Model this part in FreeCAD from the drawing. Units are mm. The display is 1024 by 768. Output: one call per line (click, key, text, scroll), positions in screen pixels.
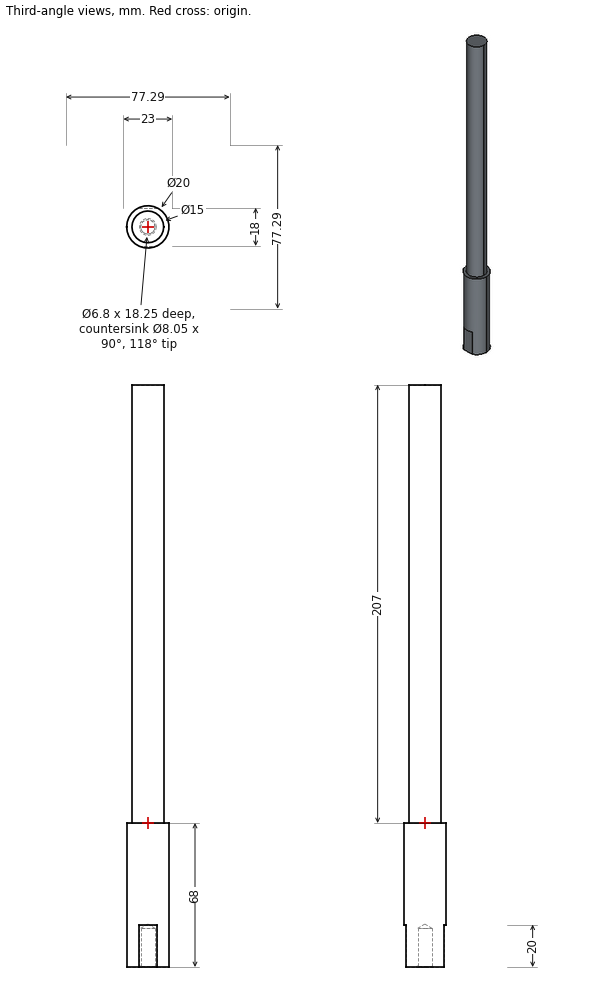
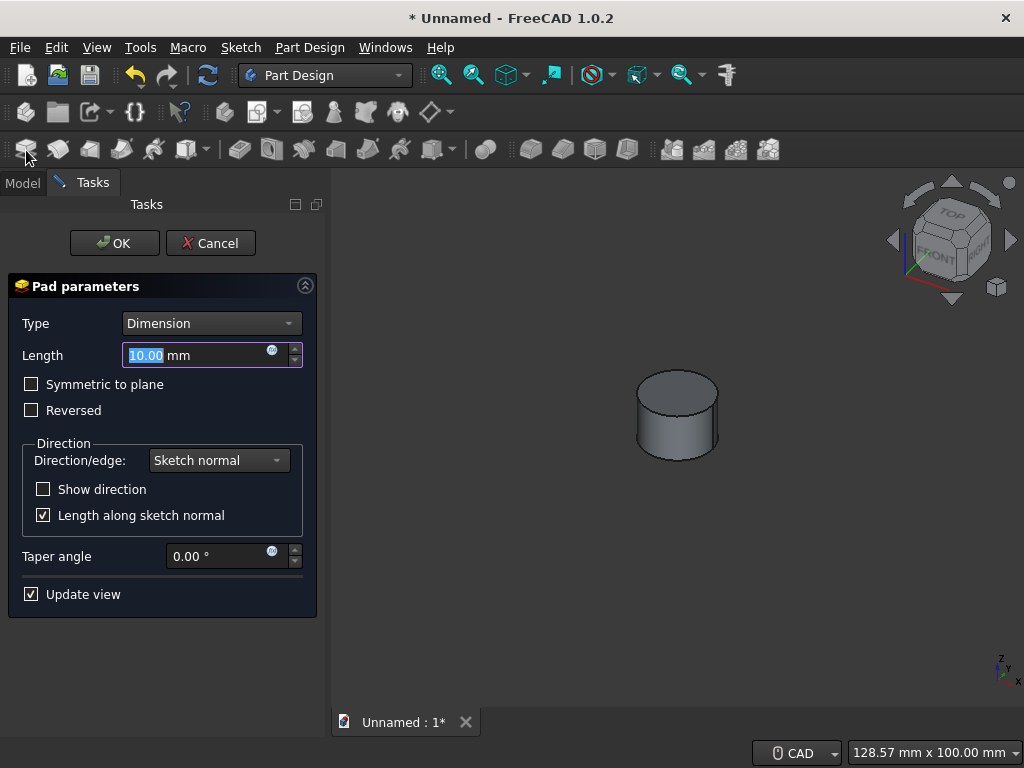
text(207)
key(Tab)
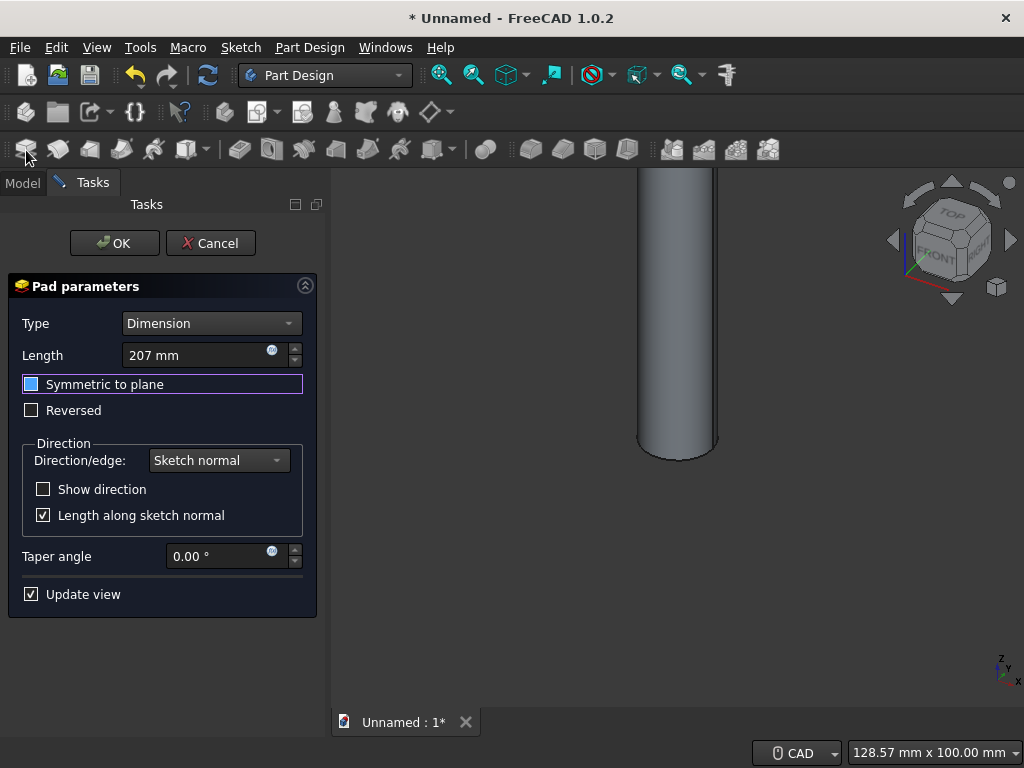
click(115, 243)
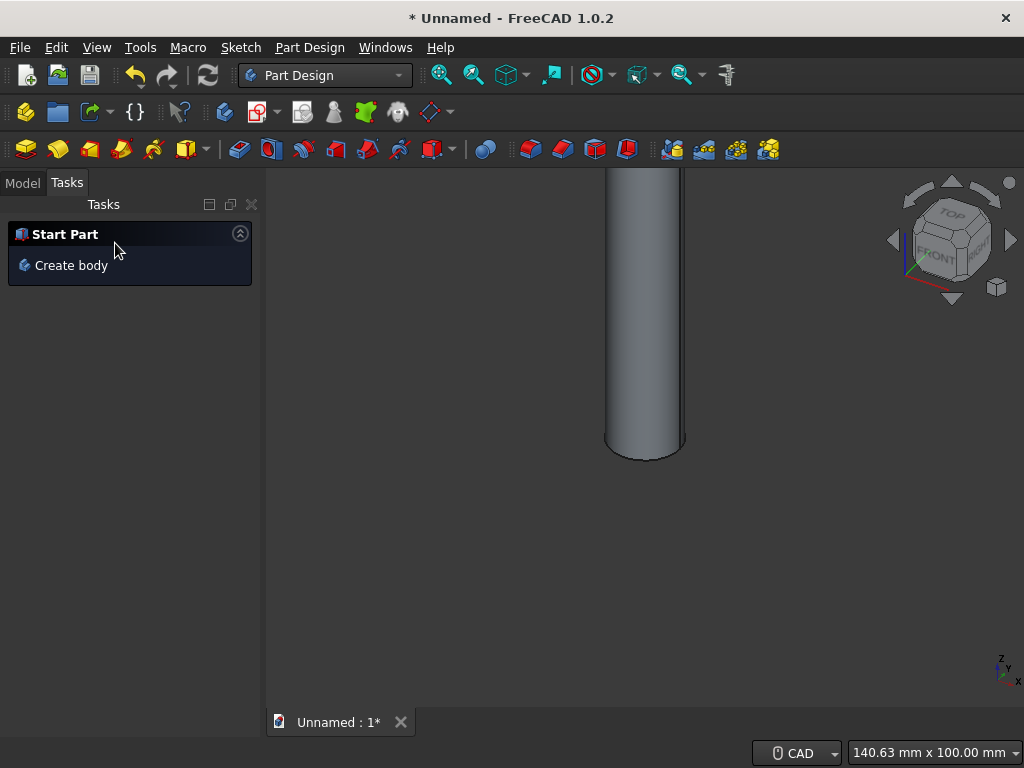
click(442, 76)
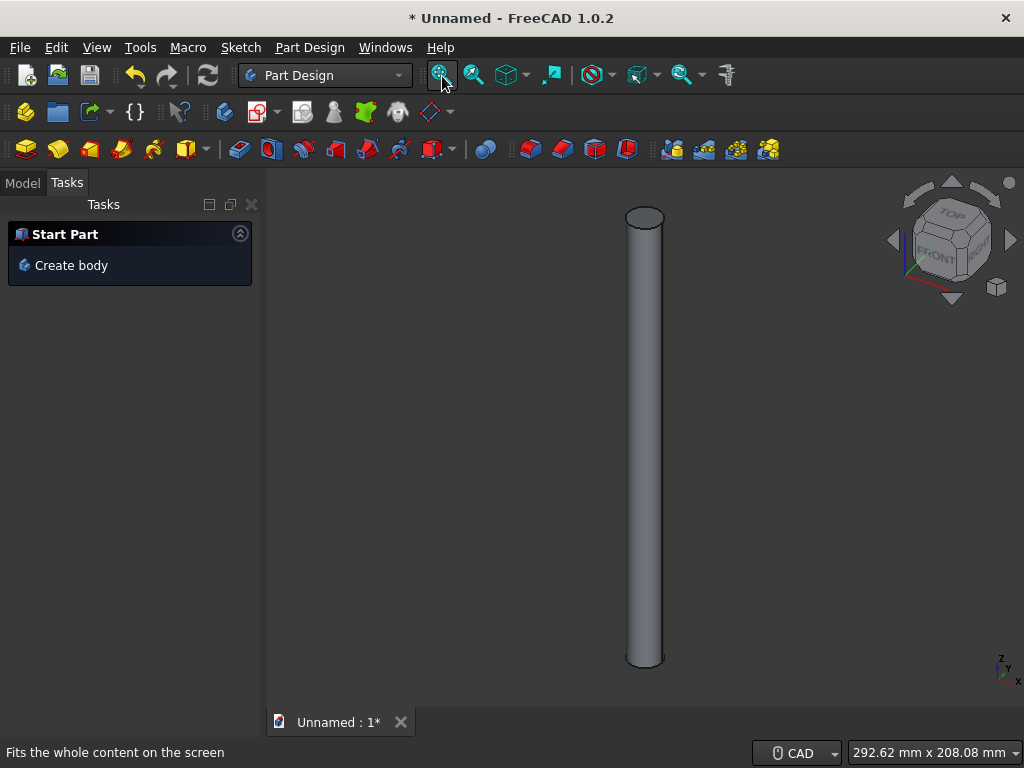
click(258, 112)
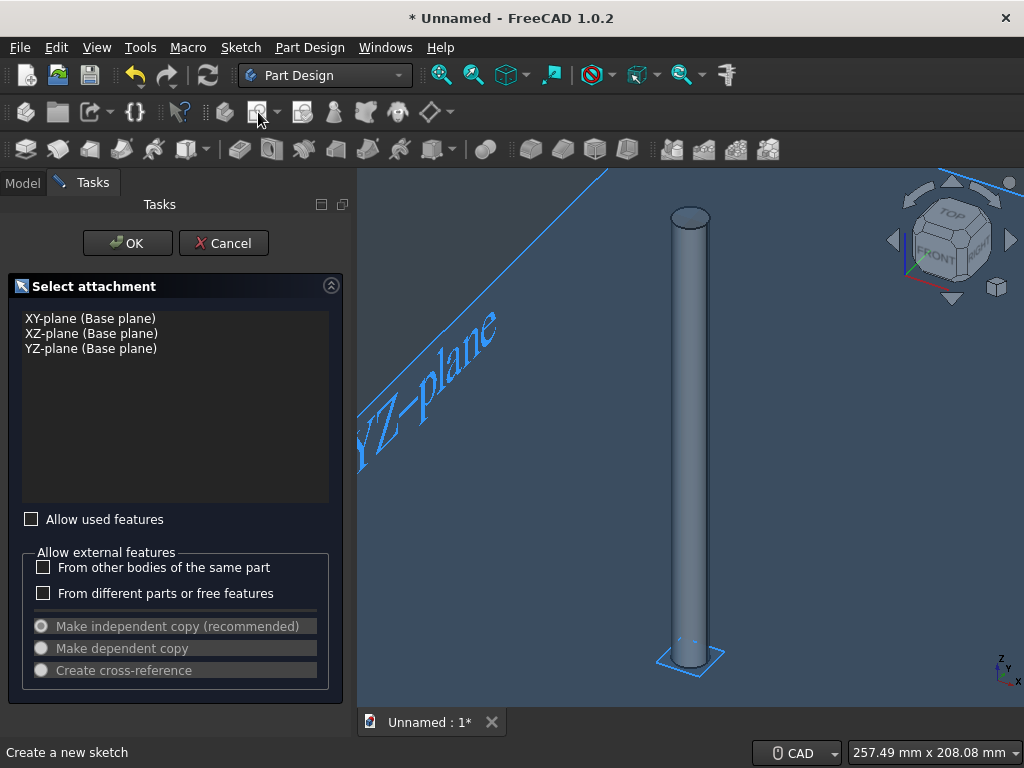
click(82, 318)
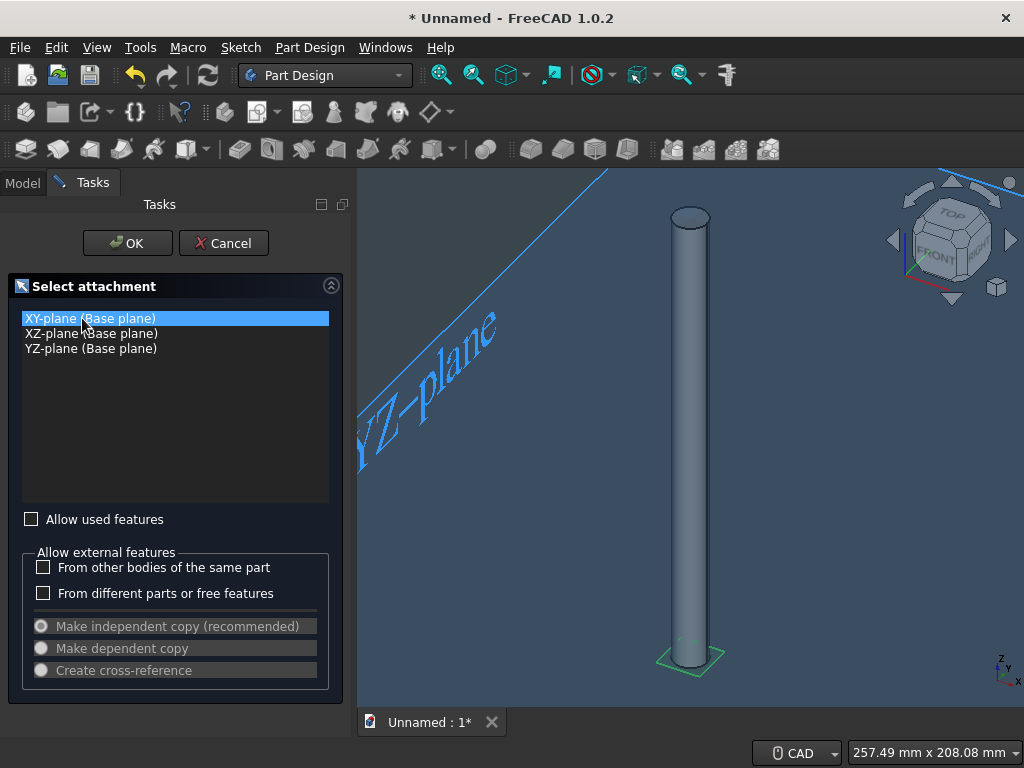
click(128, 243)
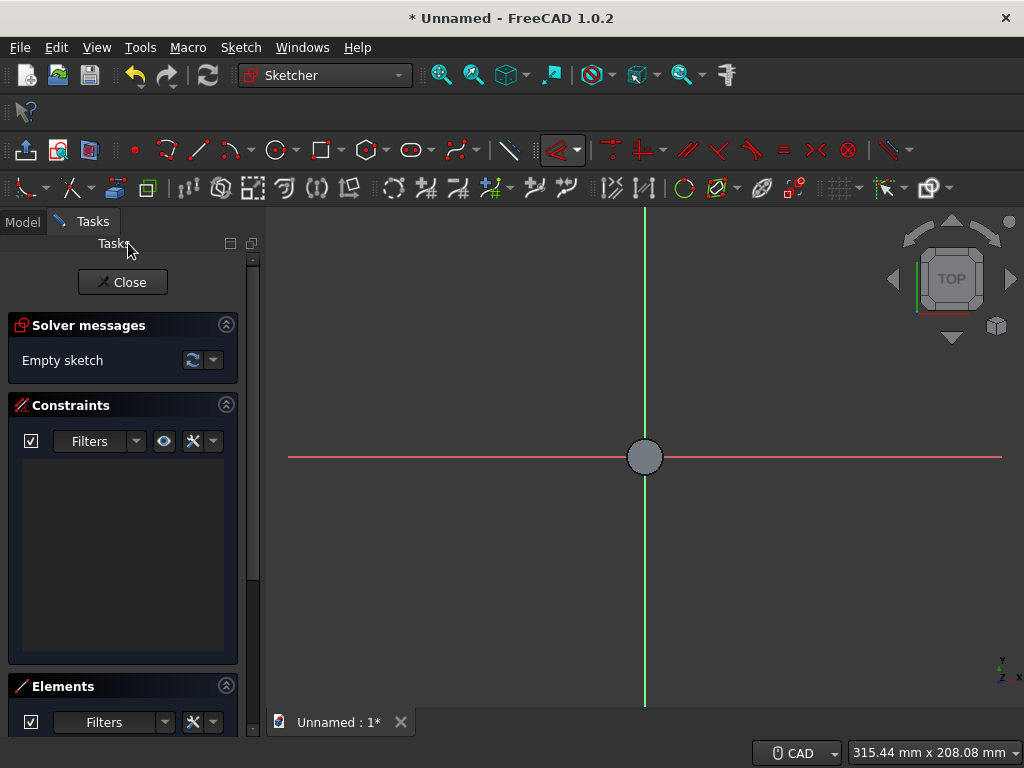
click(90, 150)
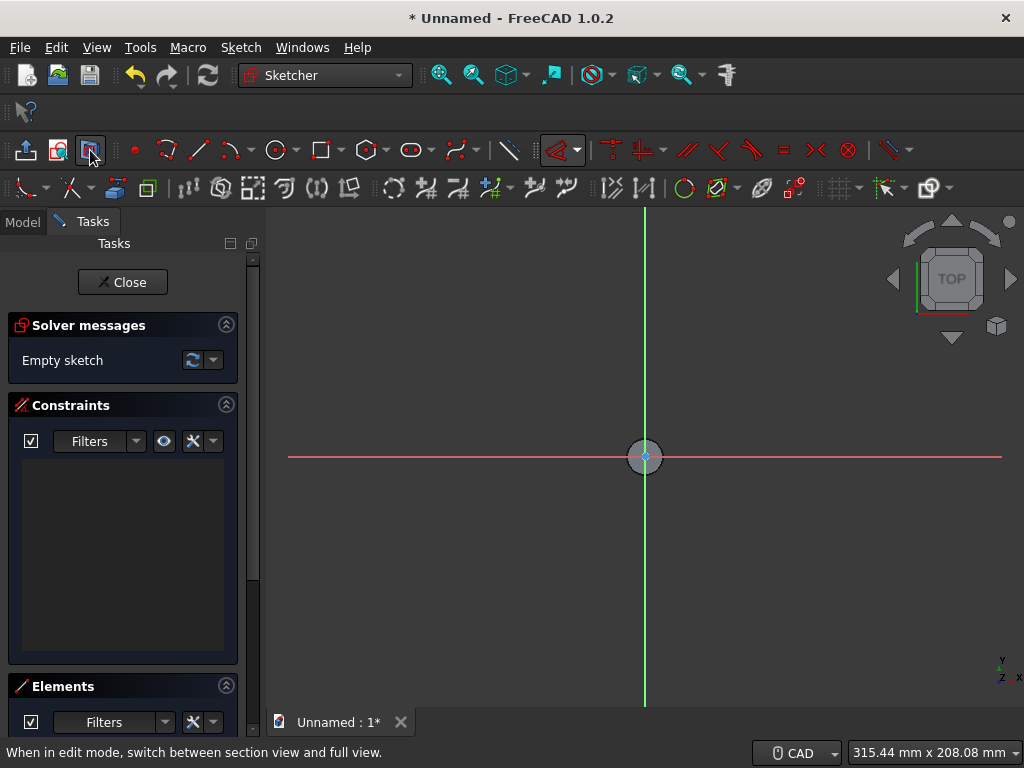
scroll(659, 457, up, 9)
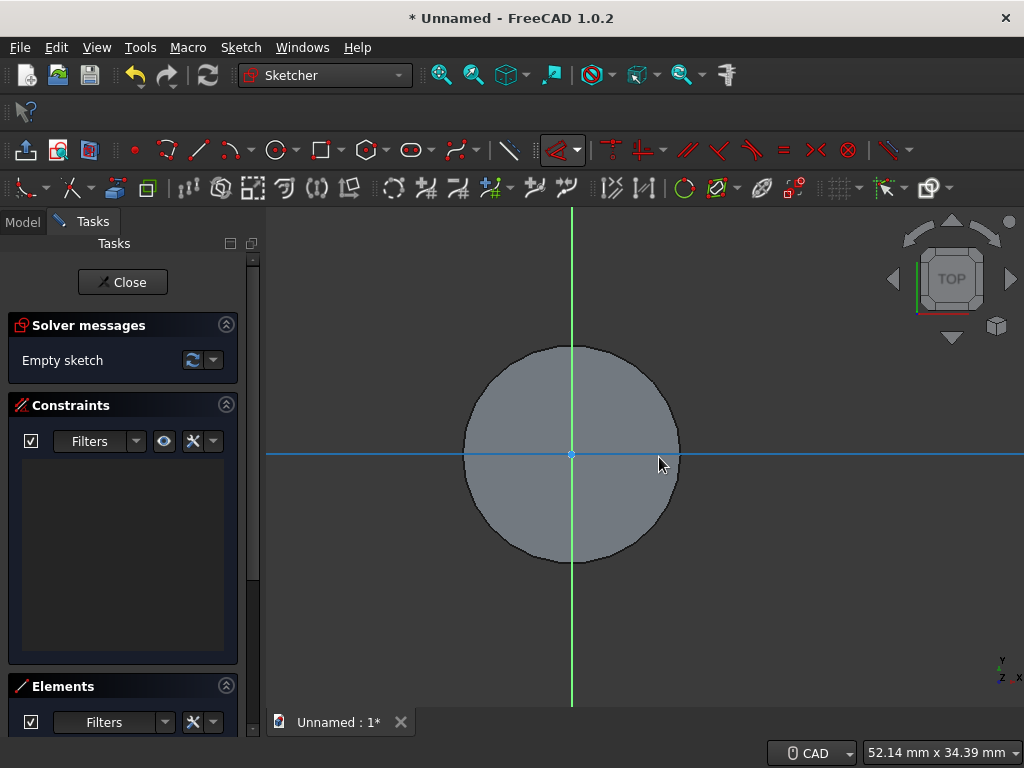
click(276, 150)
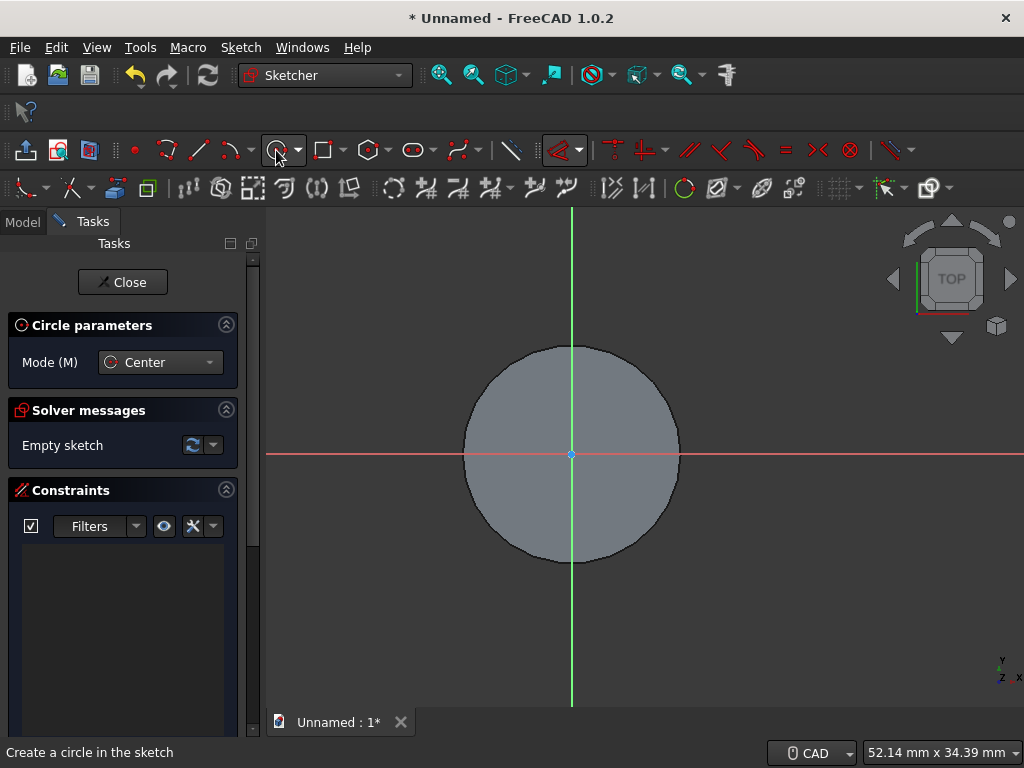
click(572, 454)
click(674, 352)
key(Escape)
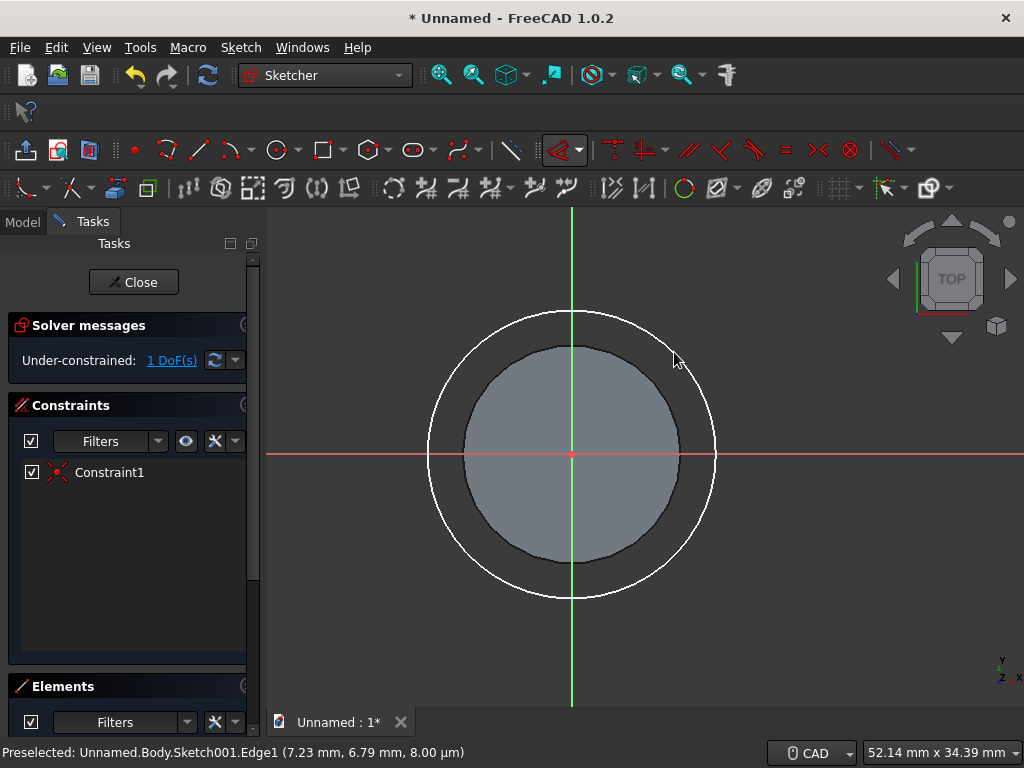
click(673, 352)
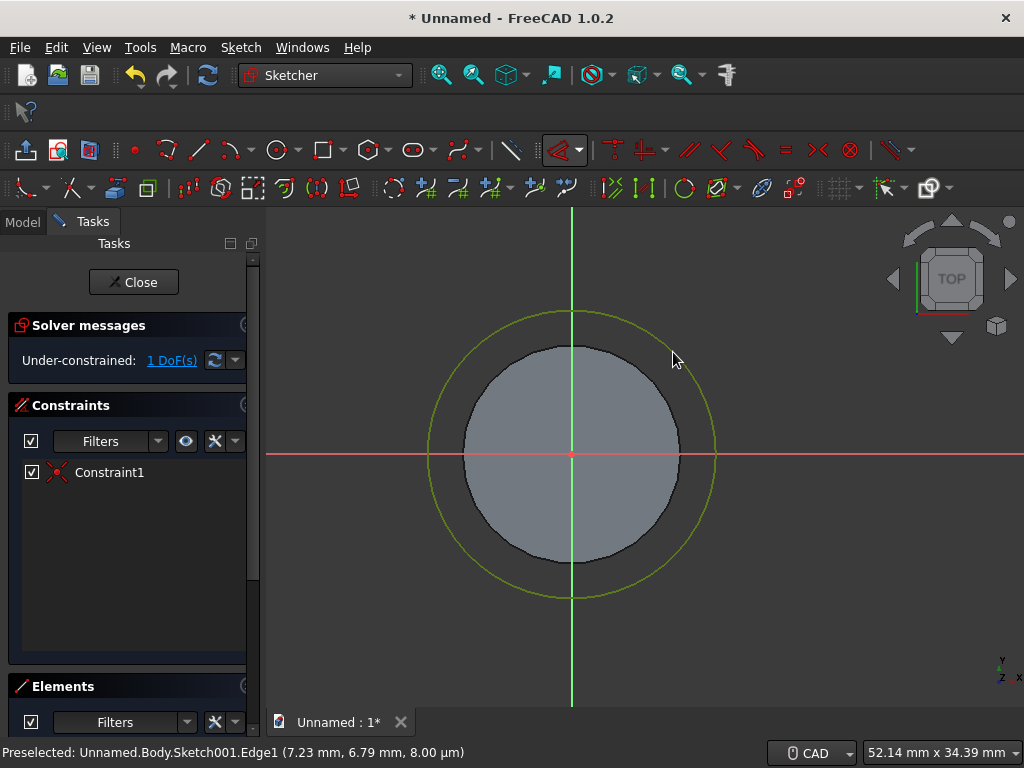
click(582, 150)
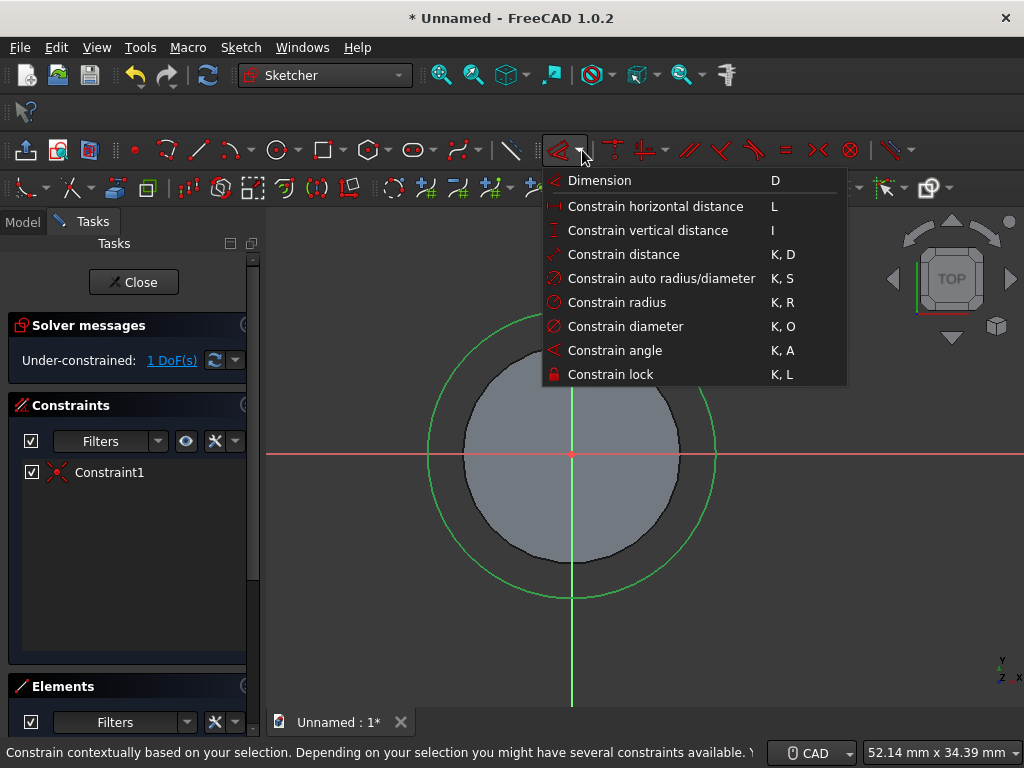
click(695, 326)